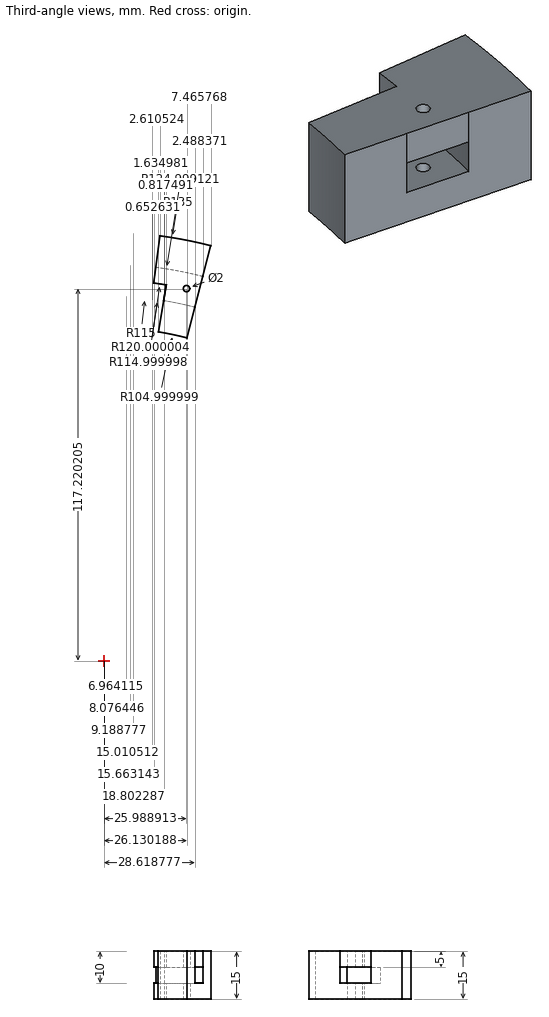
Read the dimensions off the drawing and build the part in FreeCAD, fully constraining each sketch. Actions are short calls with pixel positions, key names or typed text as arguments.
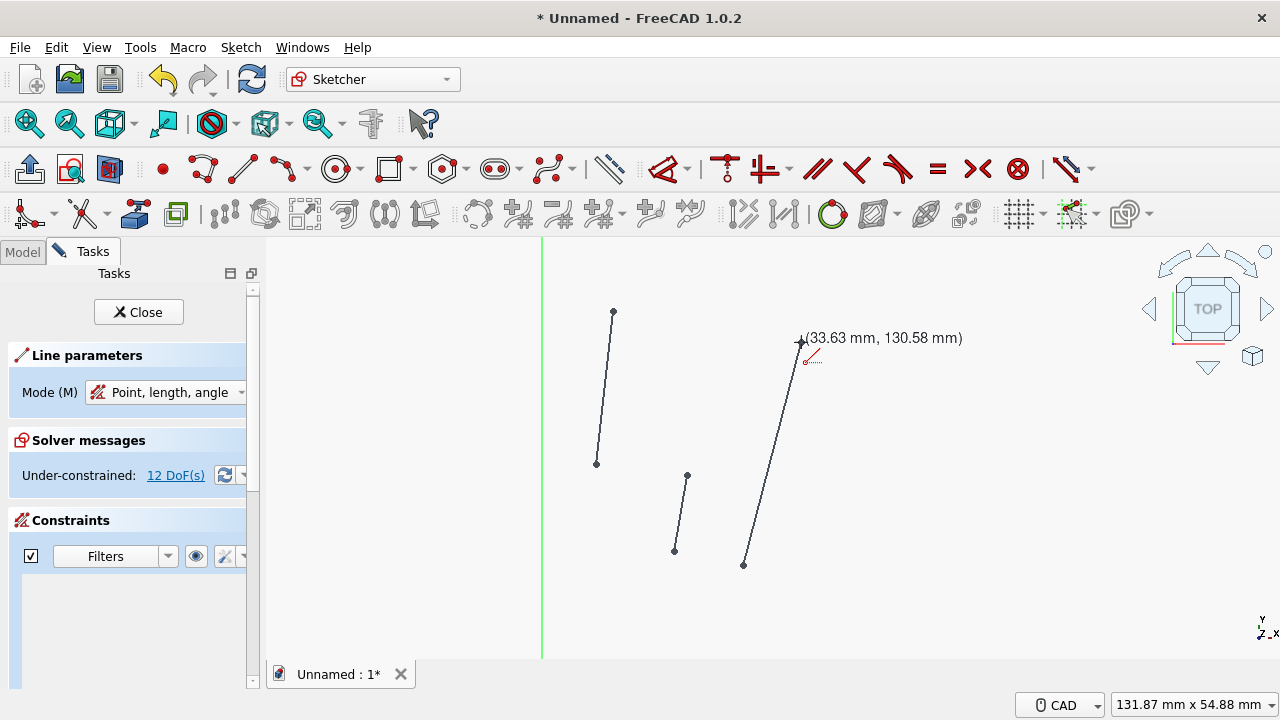
click(284, 170)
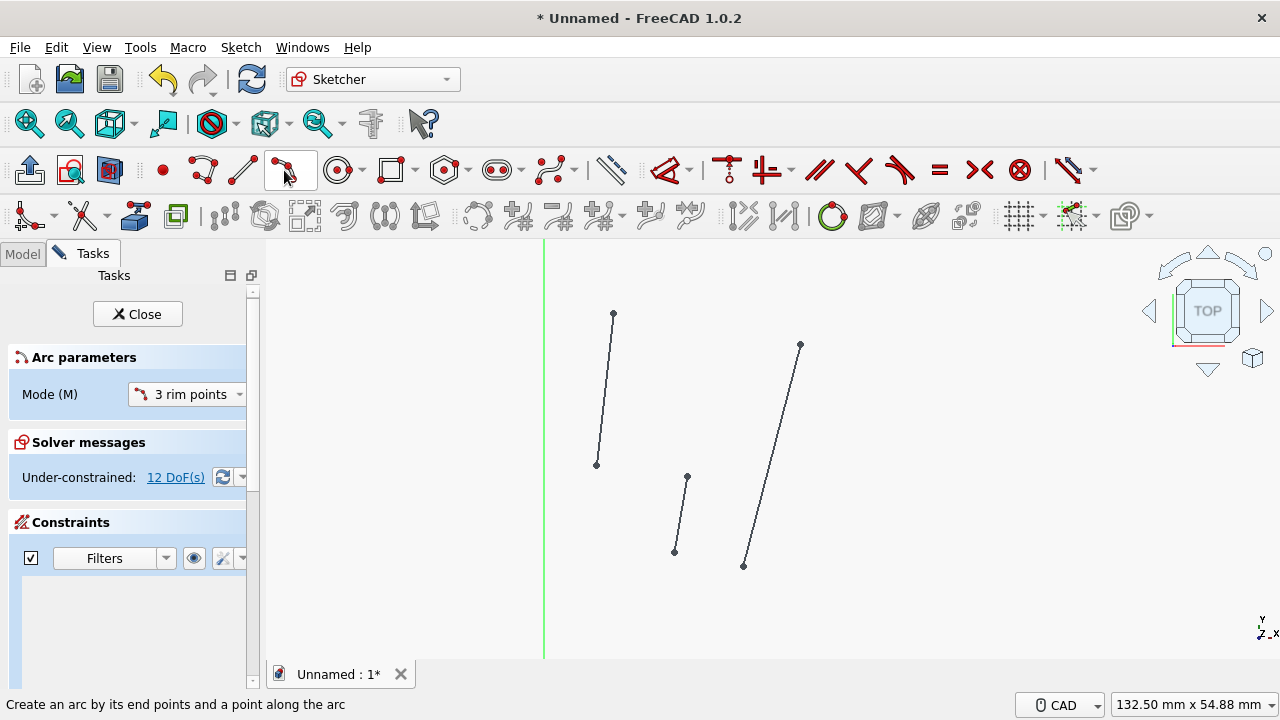
click(597, 466)
click(687, 477)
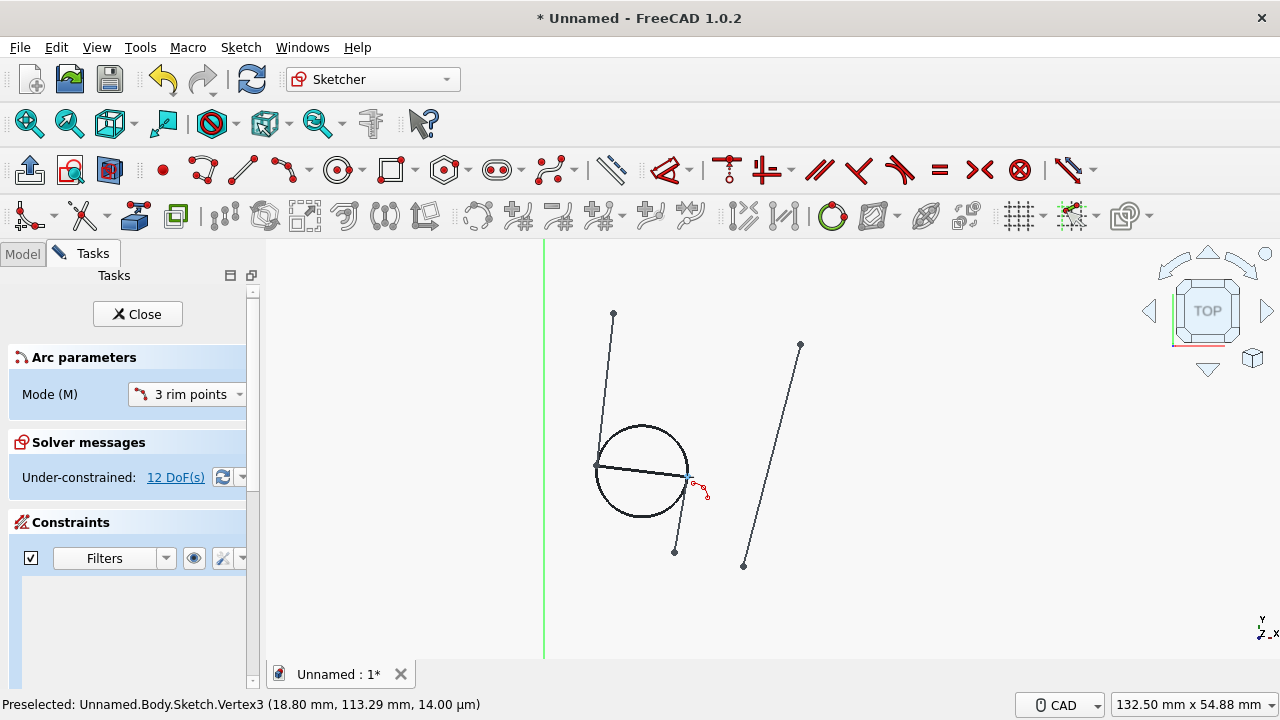
scroll(642, 469, up, 13)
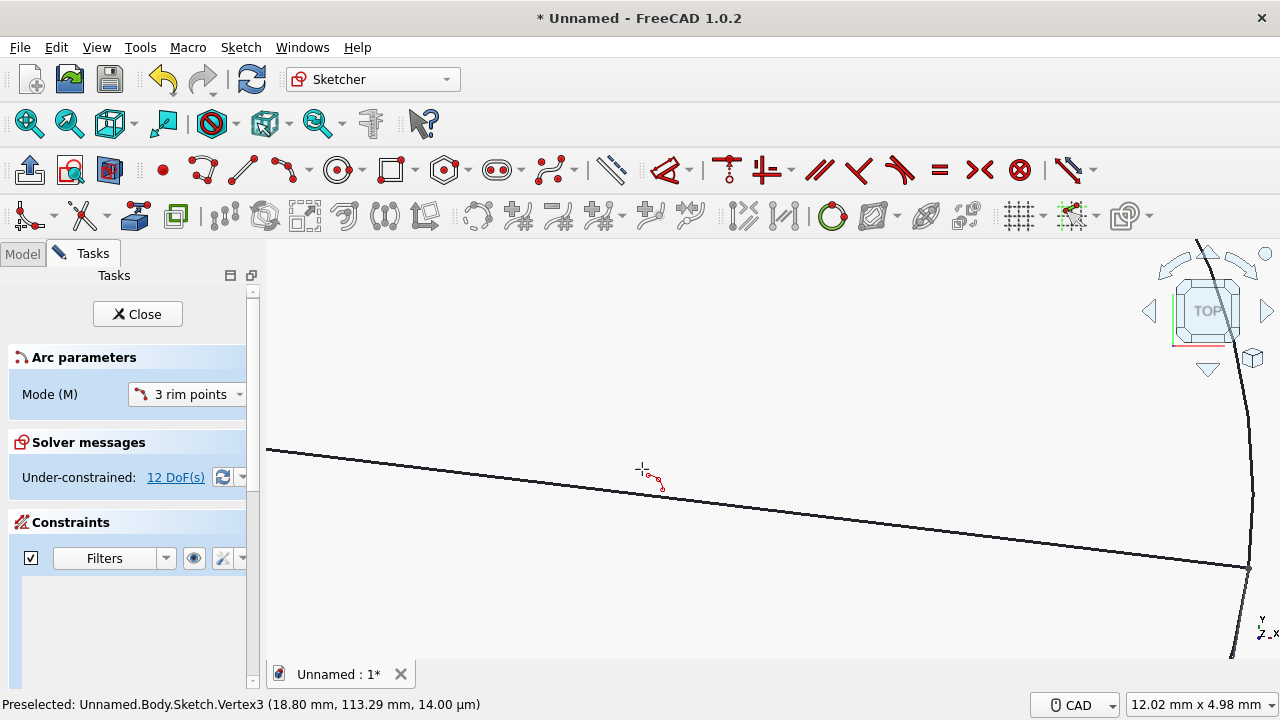
click(641, 466)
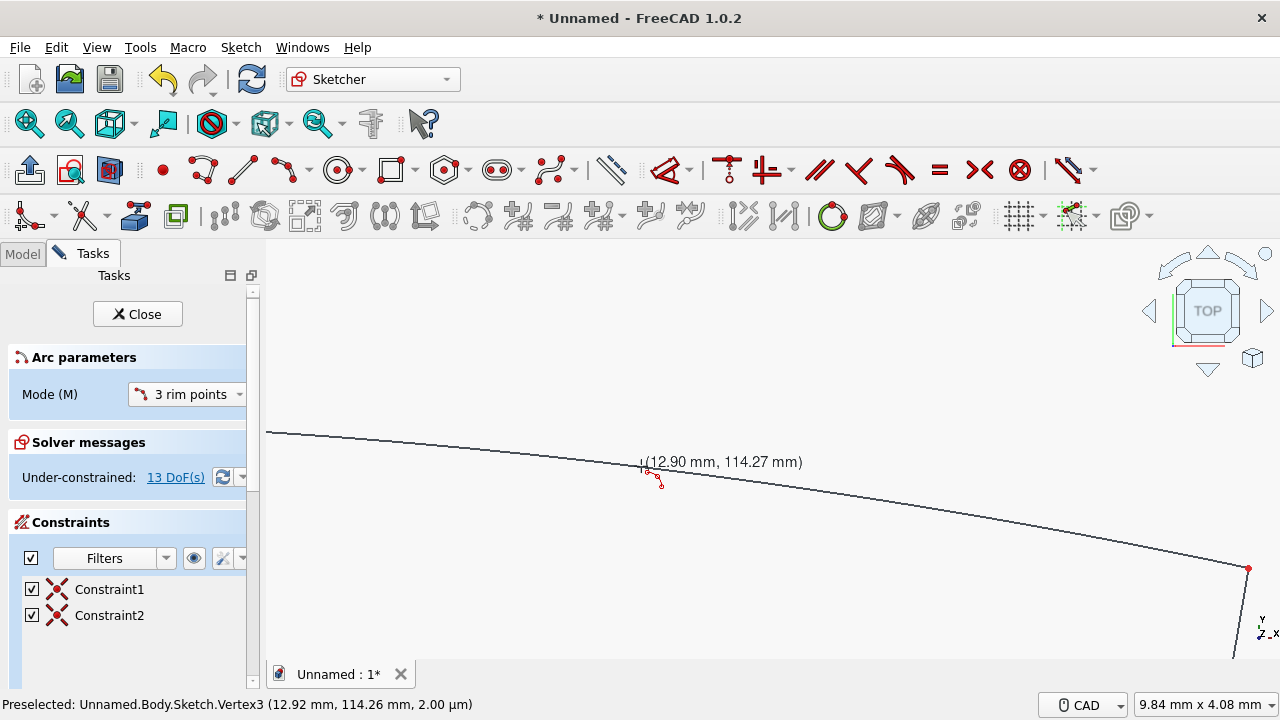
scroll(649, 480, down, 13)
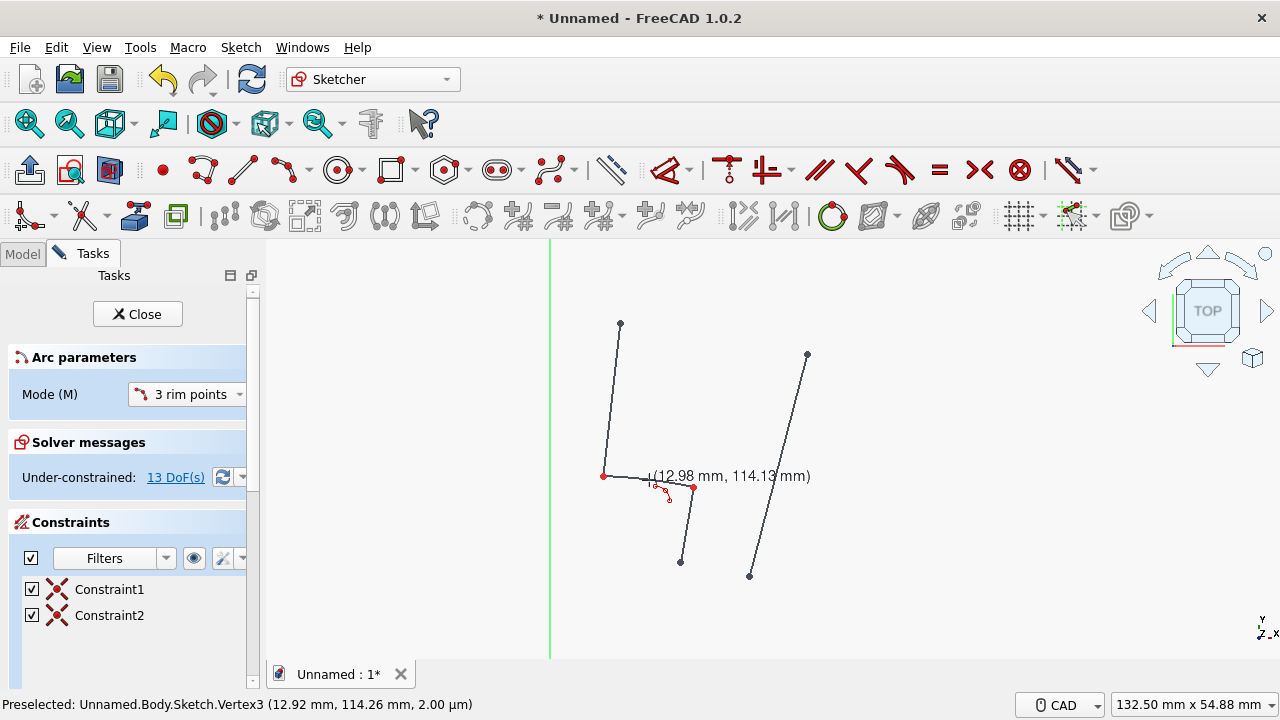
click(681, 563)
click(750, 577)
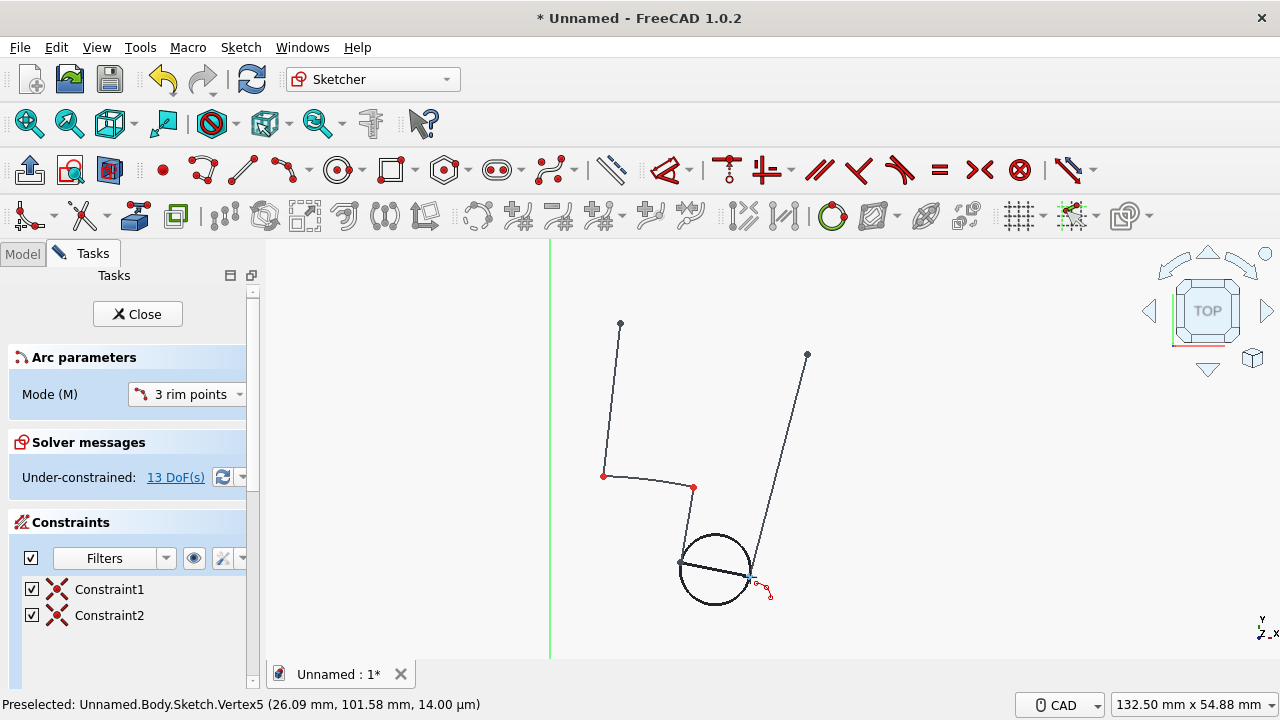
scroll(716, 568, up, 16)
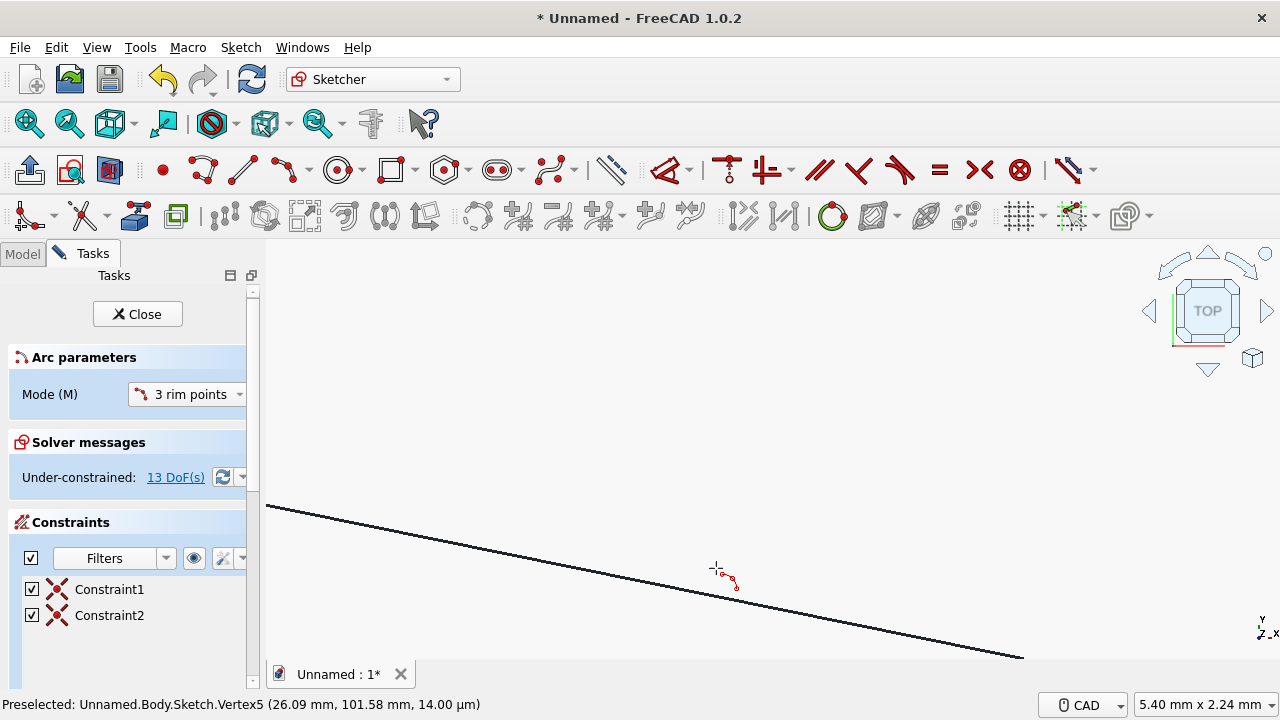
click(701, 545)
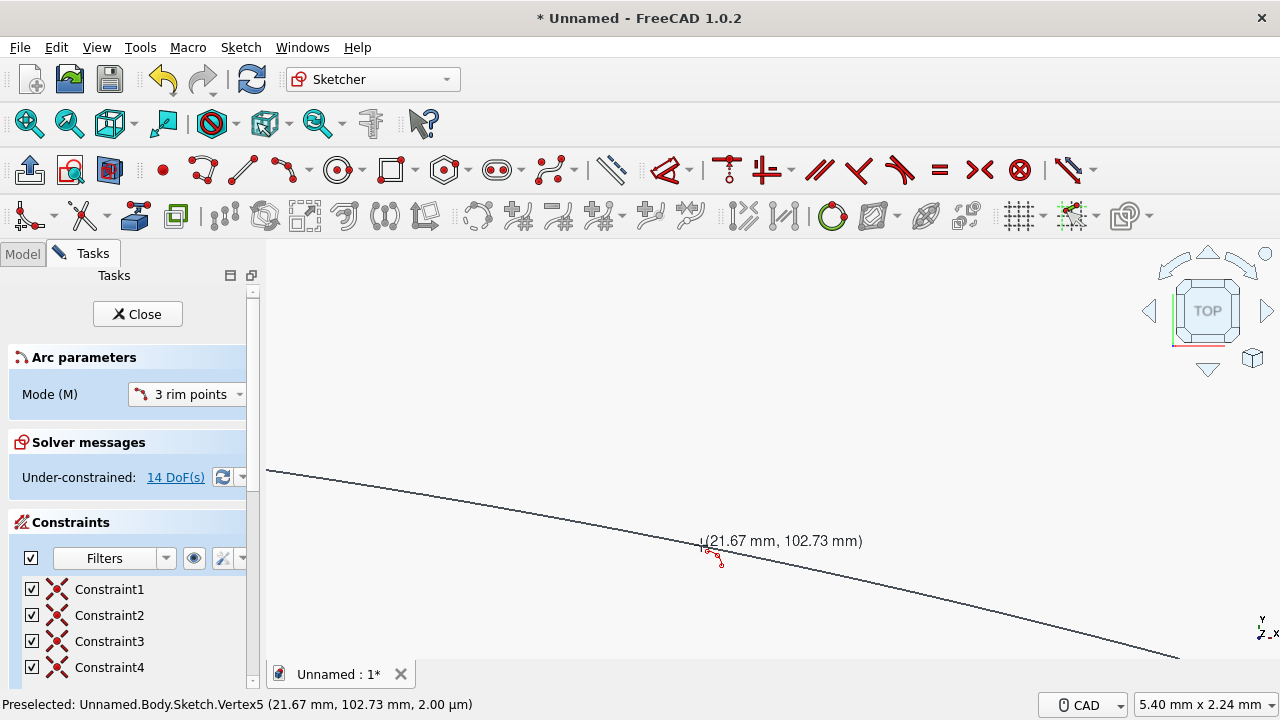
scroll(718, 596, down, 15)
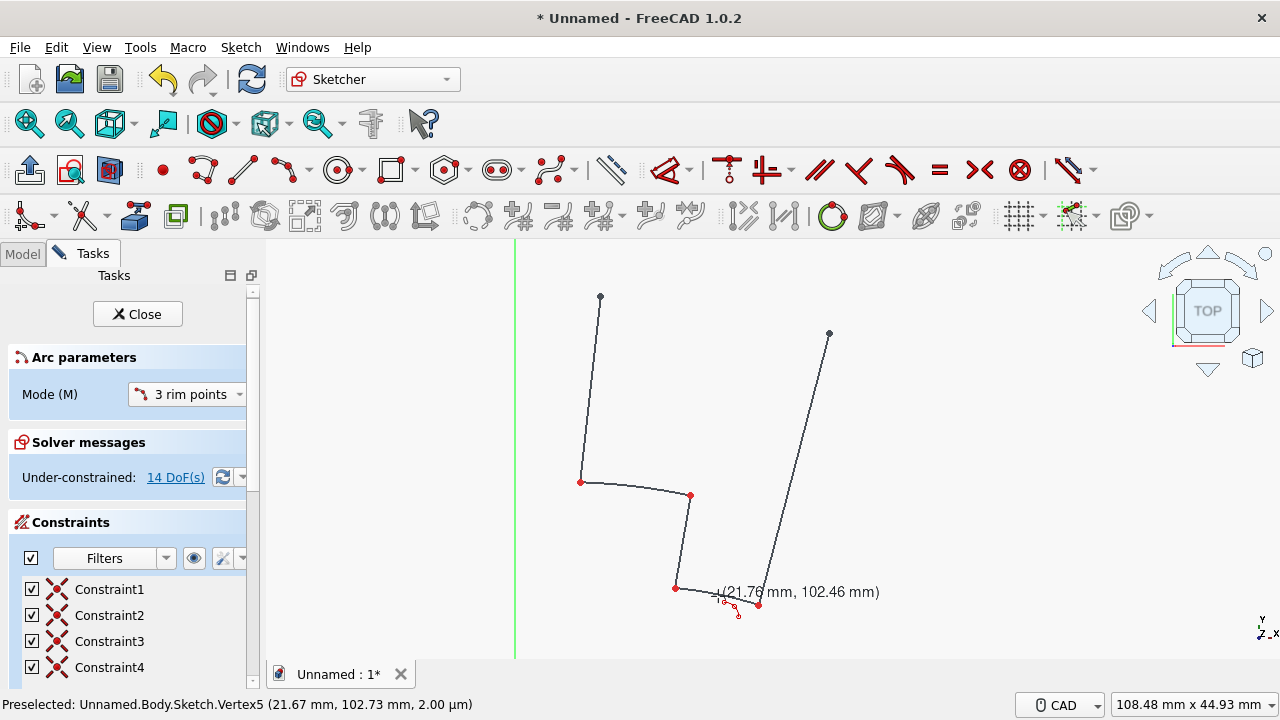
click(829, 334)
click(601, 296)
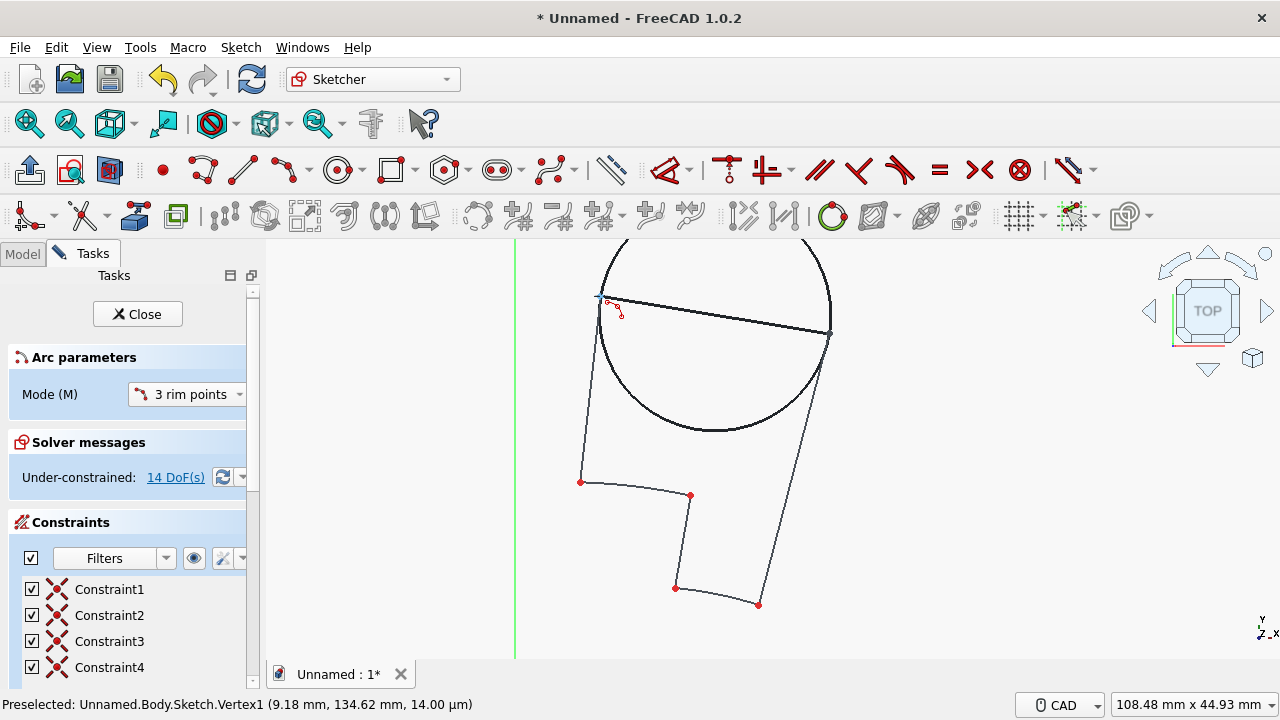
scroll(716, 309, up, 6)